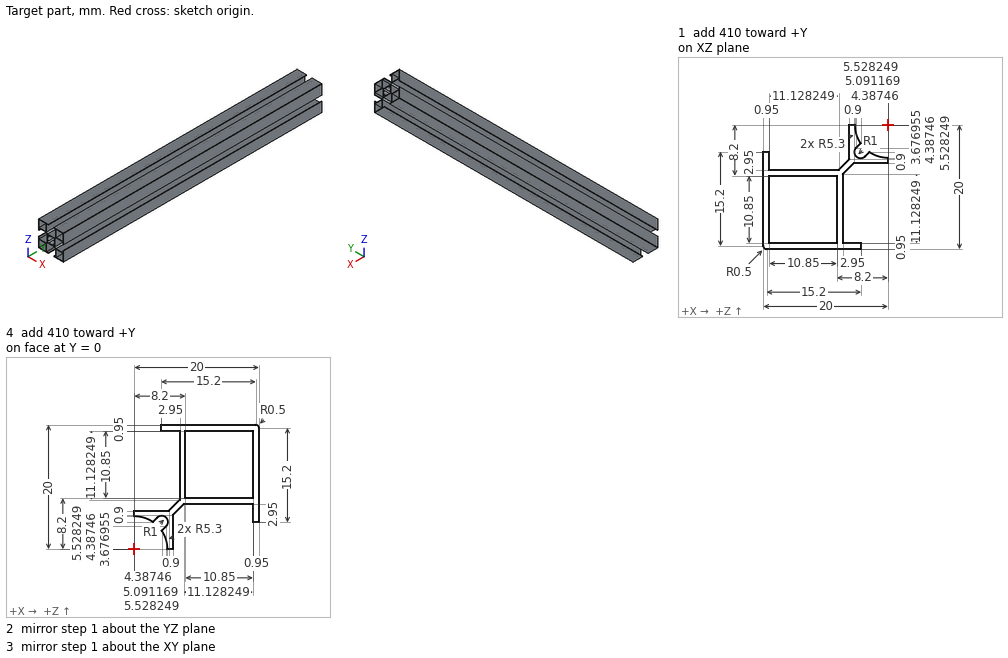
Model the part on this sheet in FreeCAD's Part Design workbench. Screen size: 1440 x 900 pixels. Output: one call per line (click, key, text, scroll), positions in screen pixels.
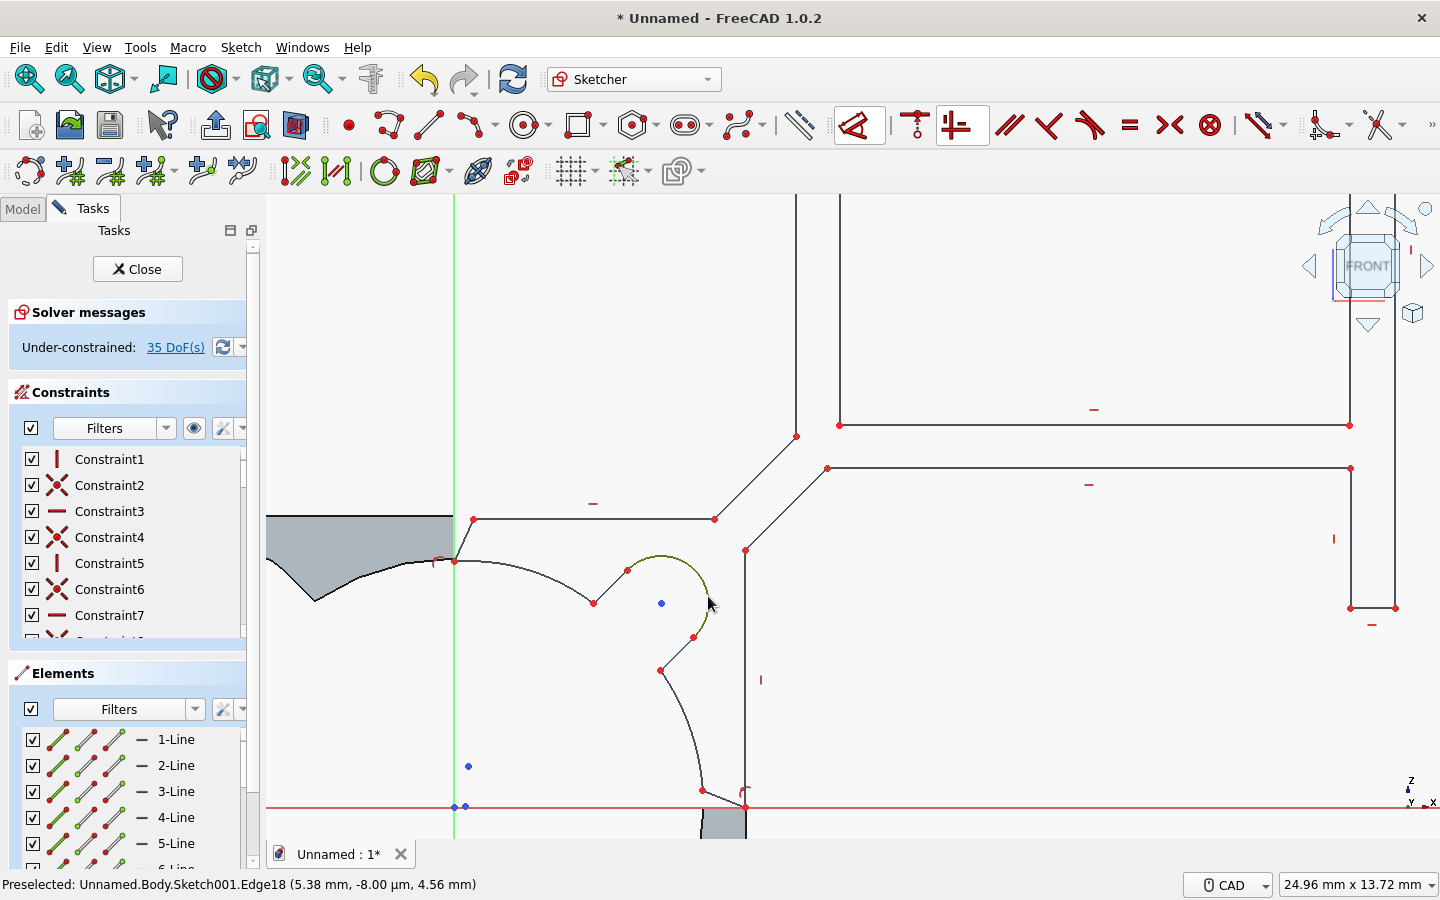
click(1090, 126)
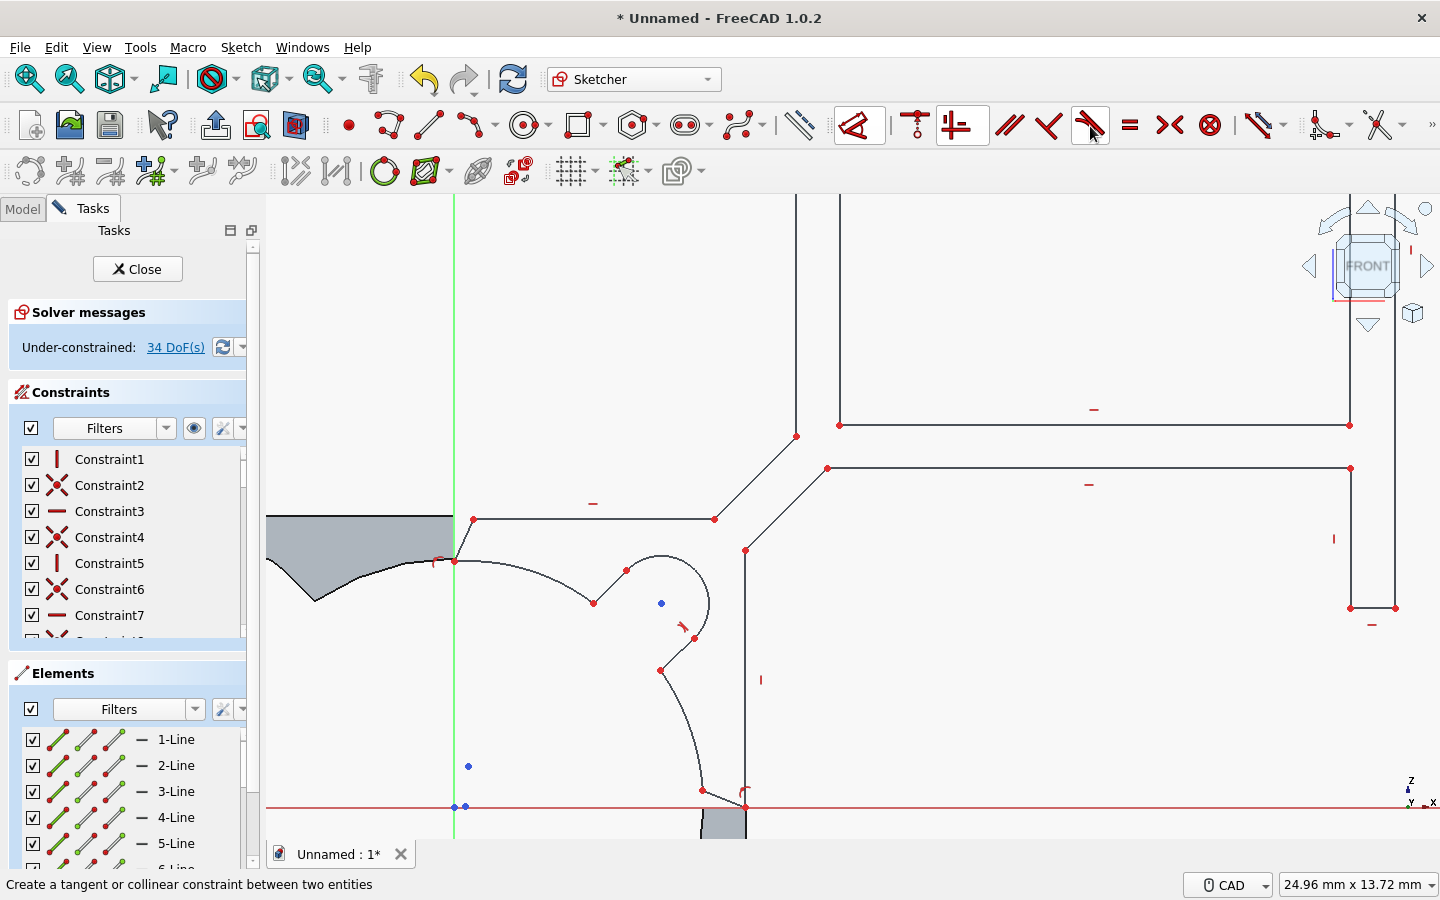
click(617, 581)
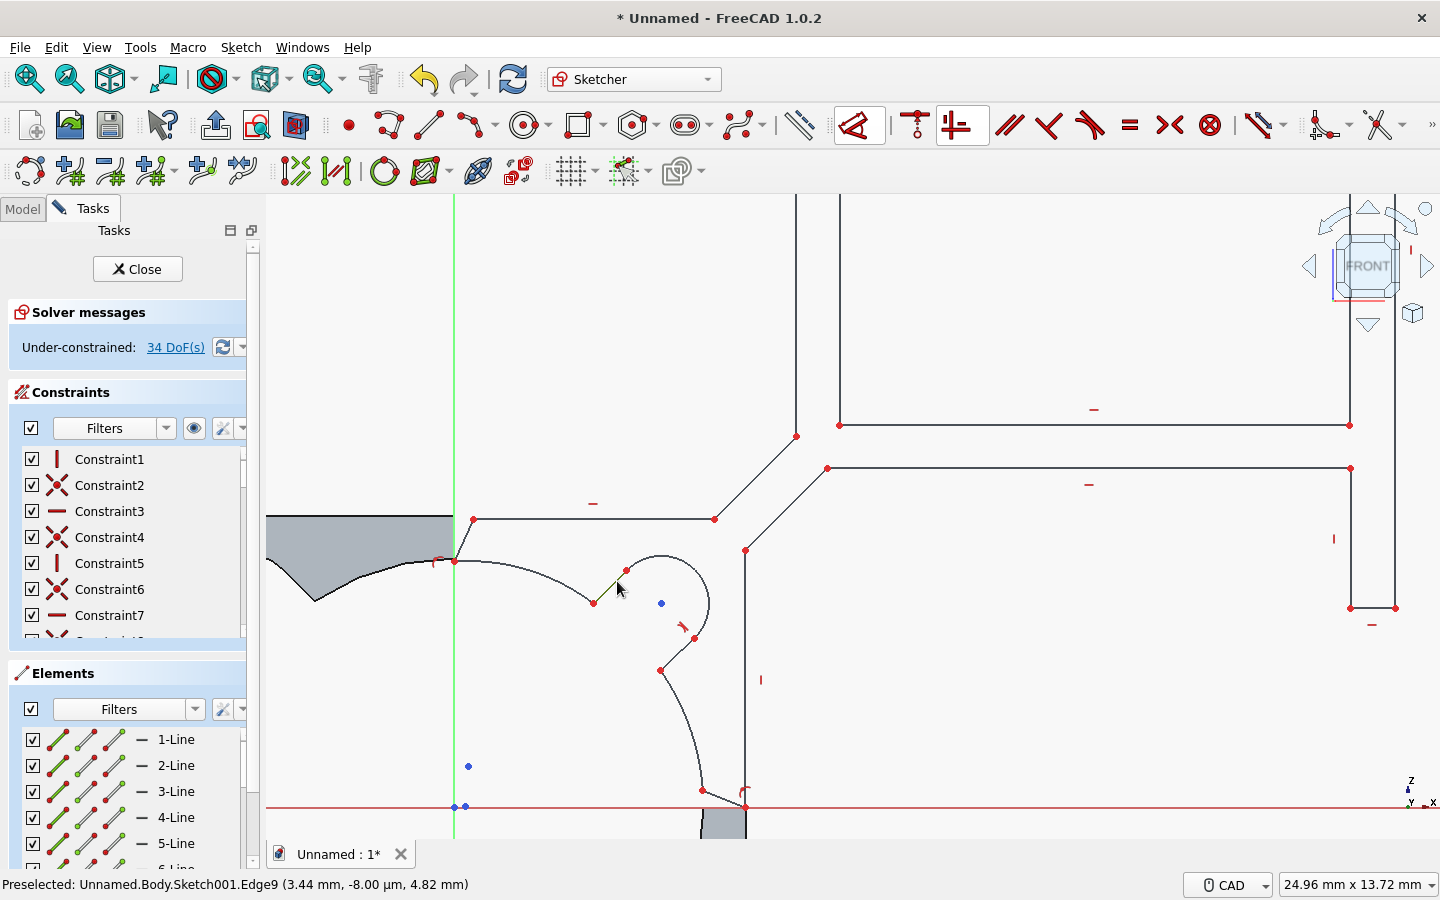
click(708, 597)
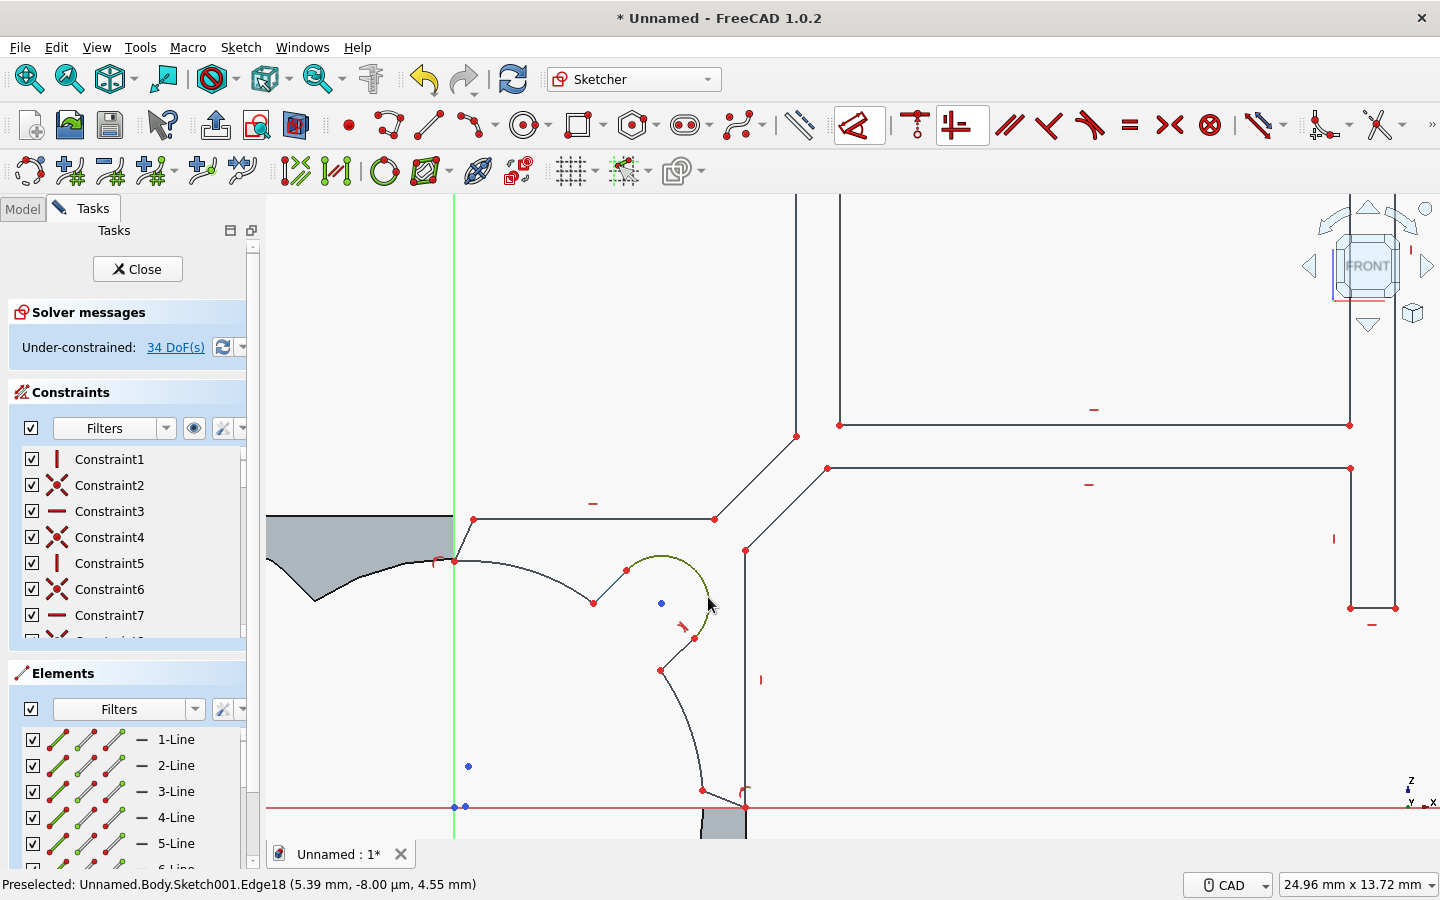
key(t)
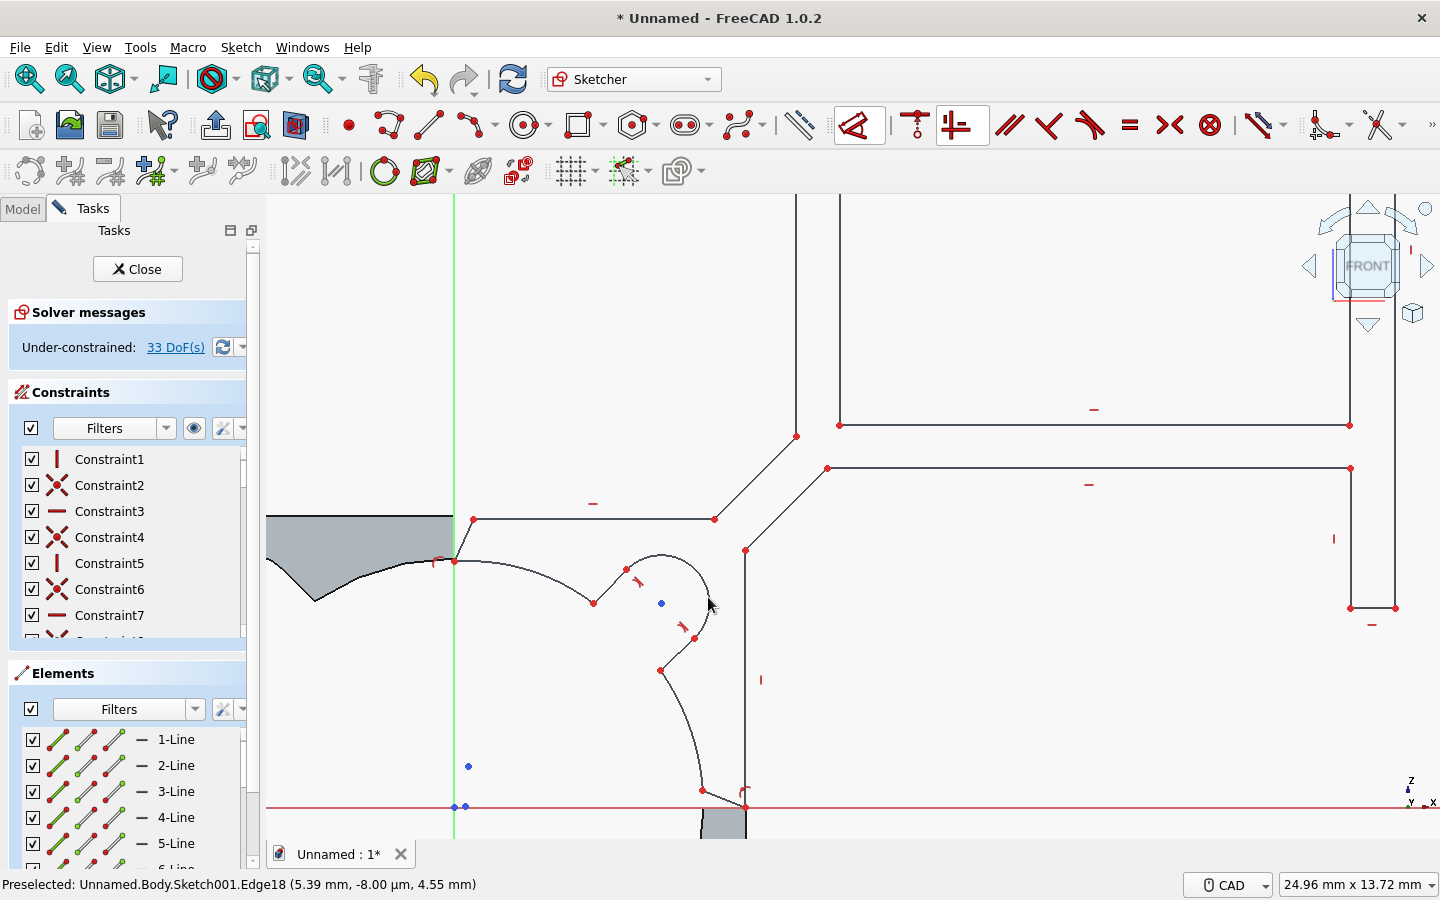
scroll(670, 663, down, 4)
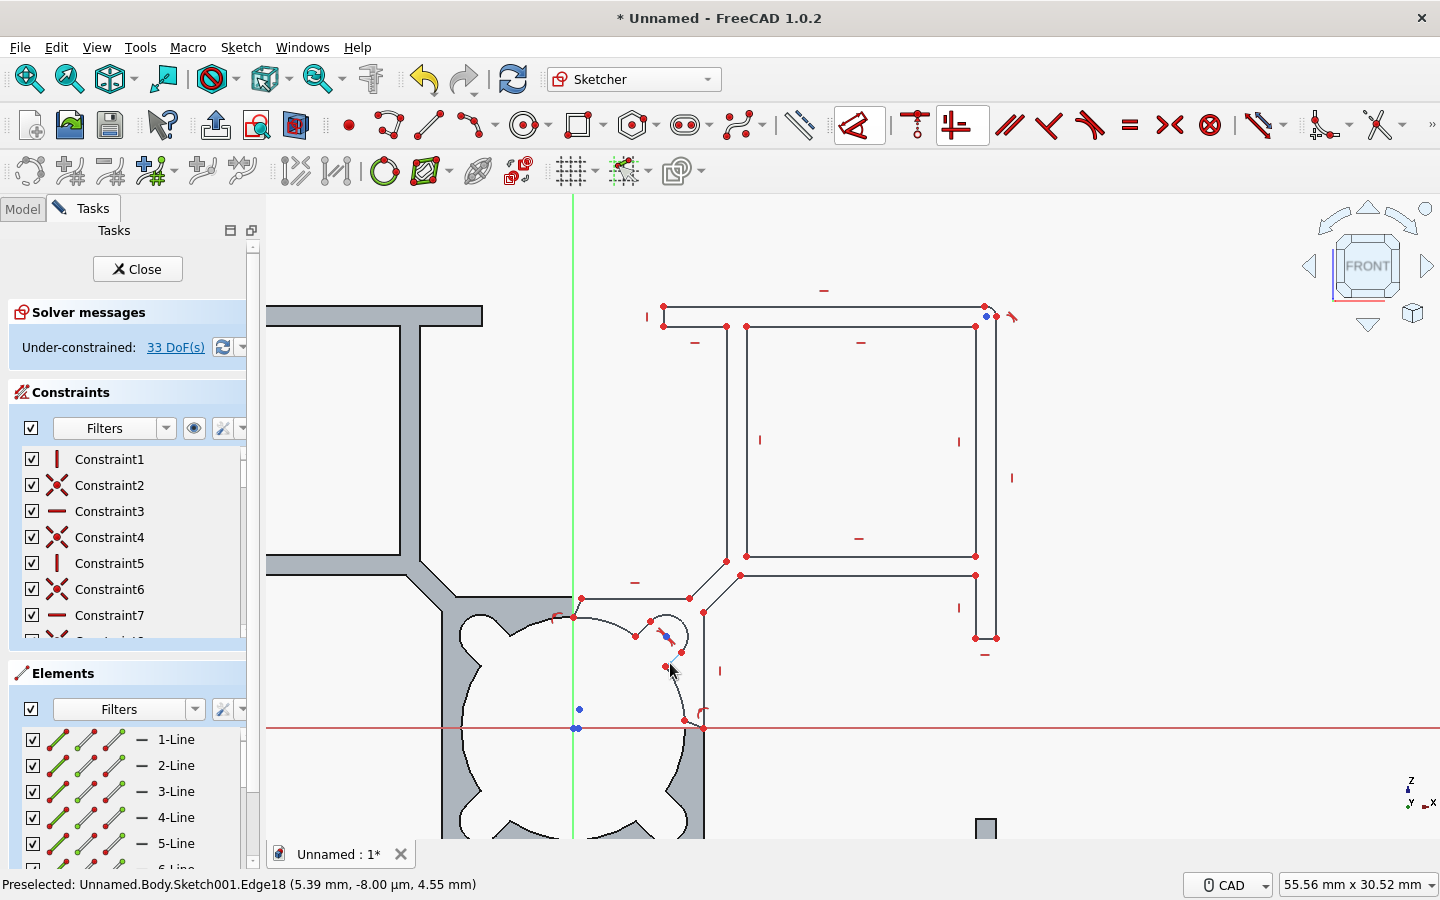
click(760, 307)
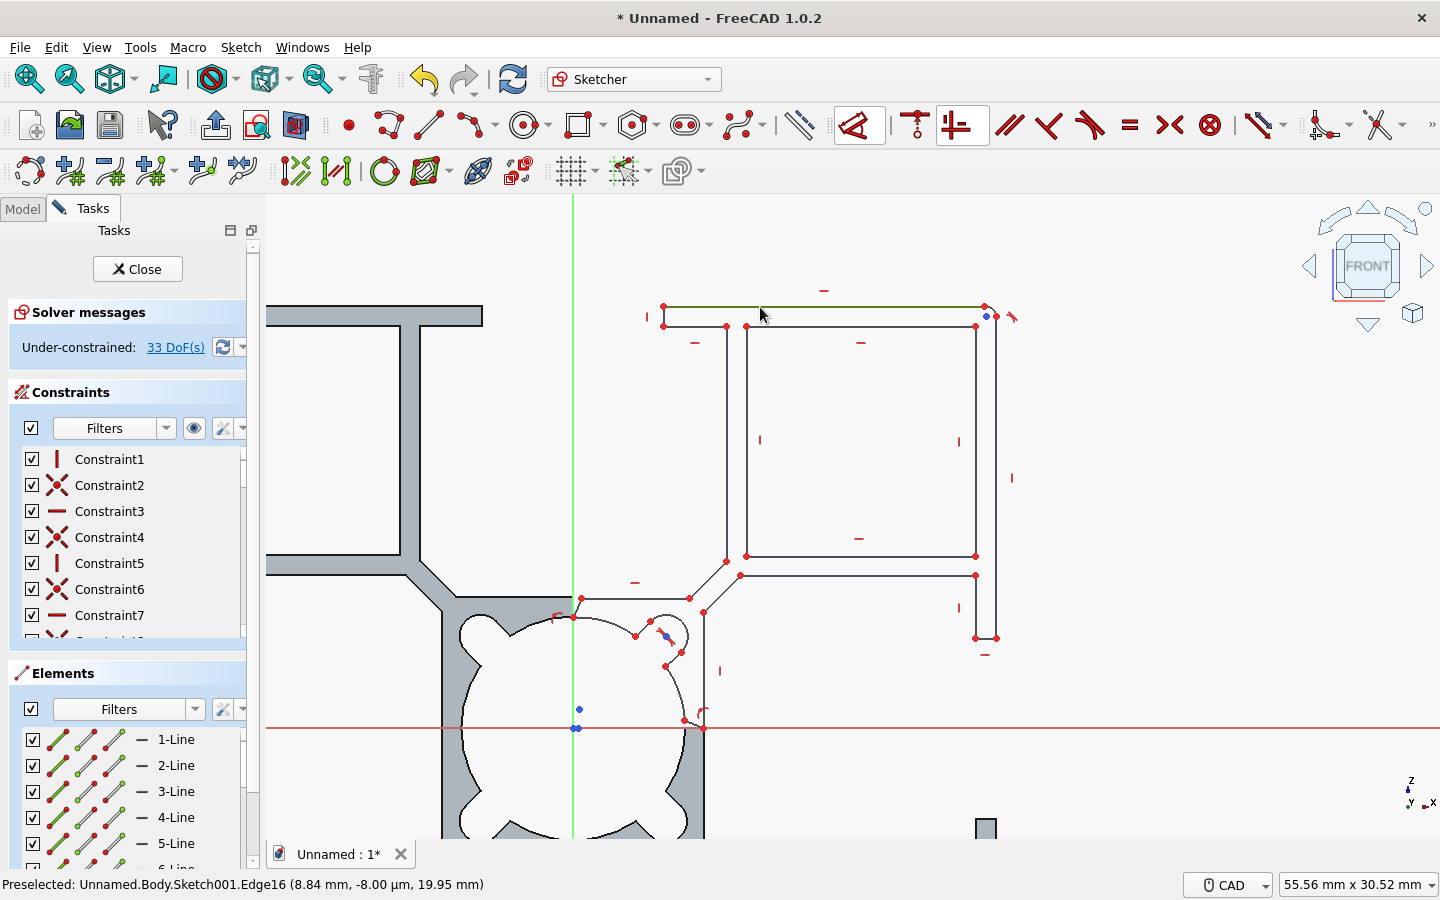
scroll(993, 309, up, 3)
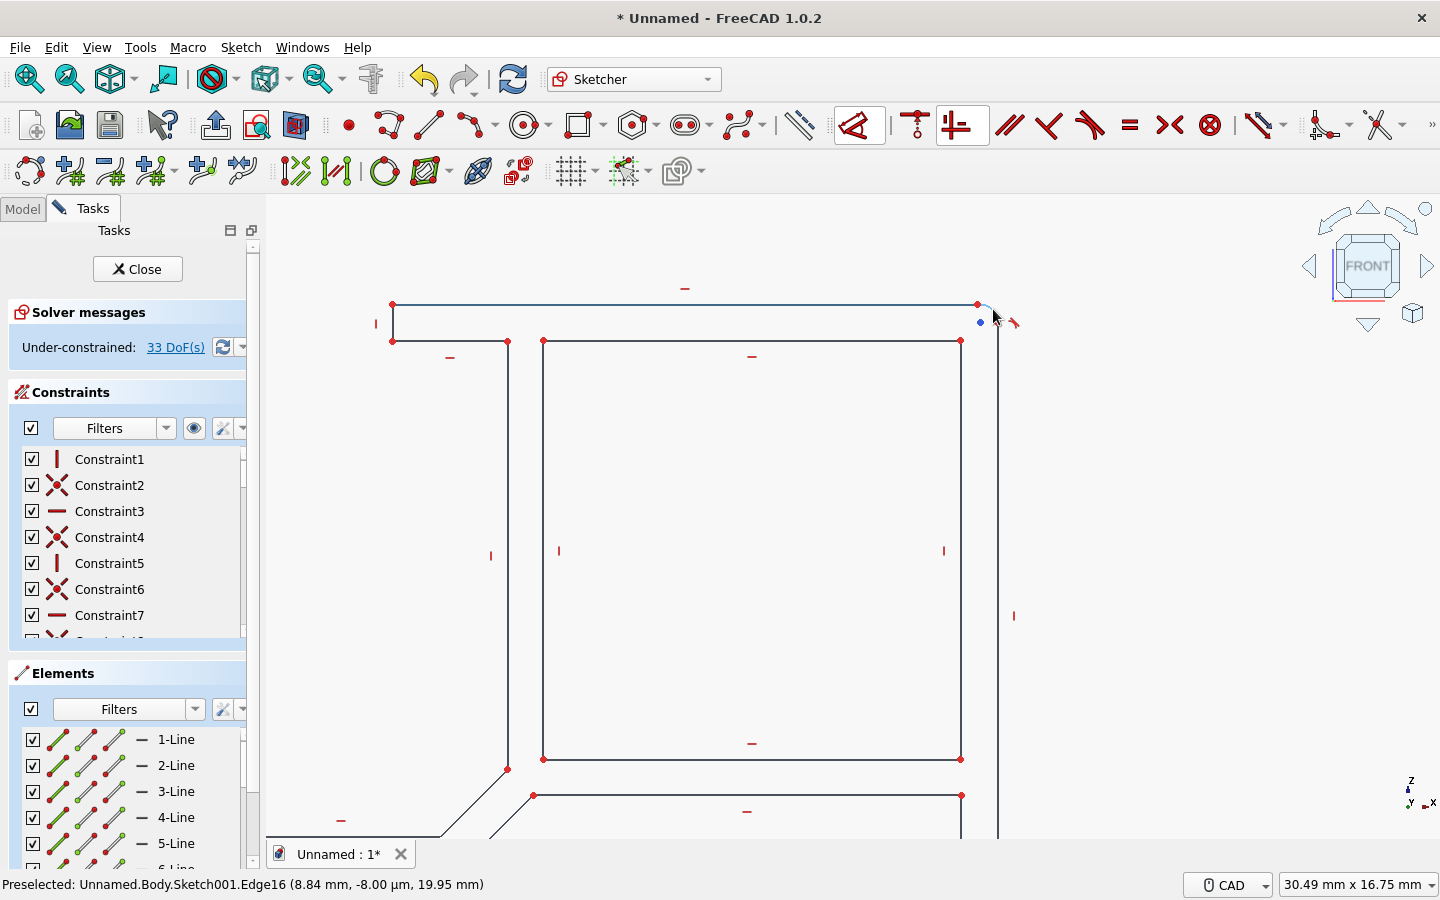
click(992, 309)